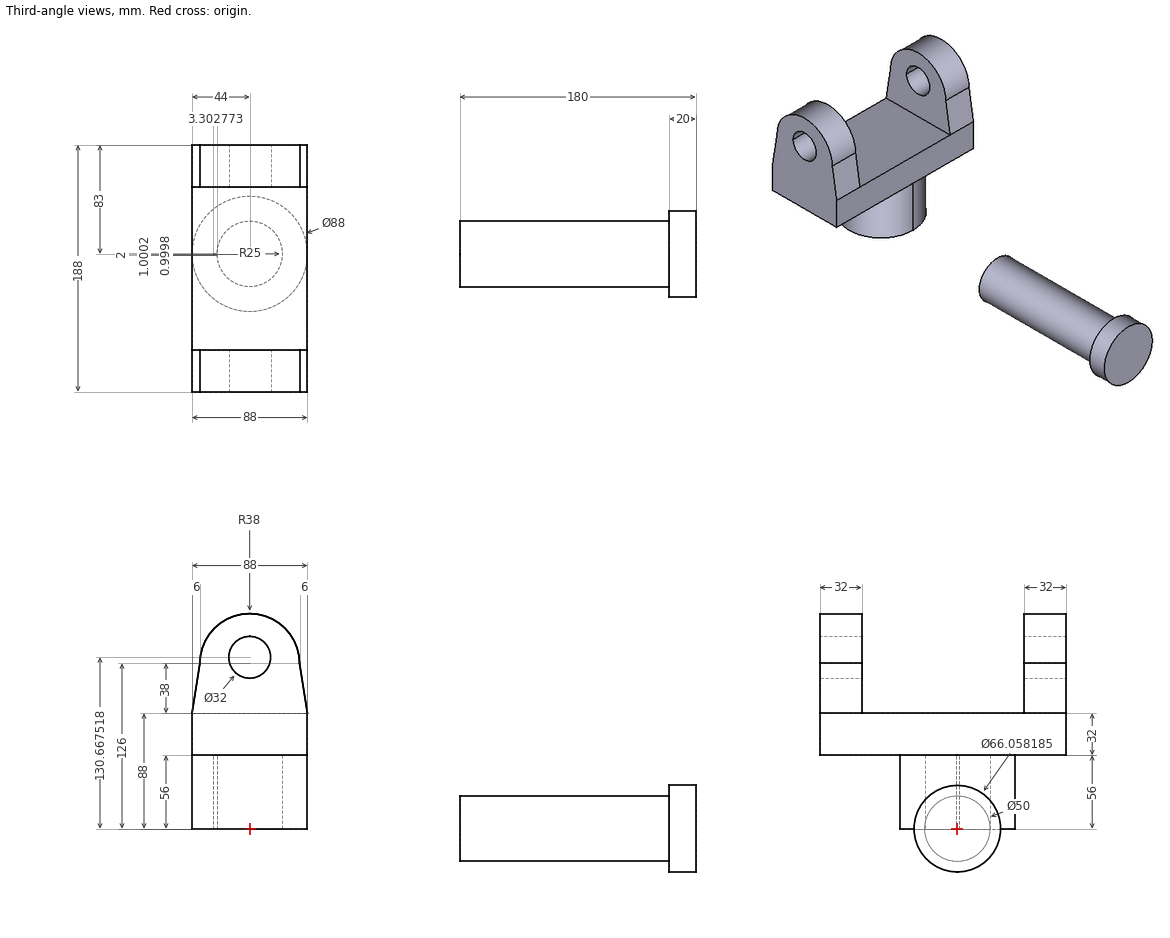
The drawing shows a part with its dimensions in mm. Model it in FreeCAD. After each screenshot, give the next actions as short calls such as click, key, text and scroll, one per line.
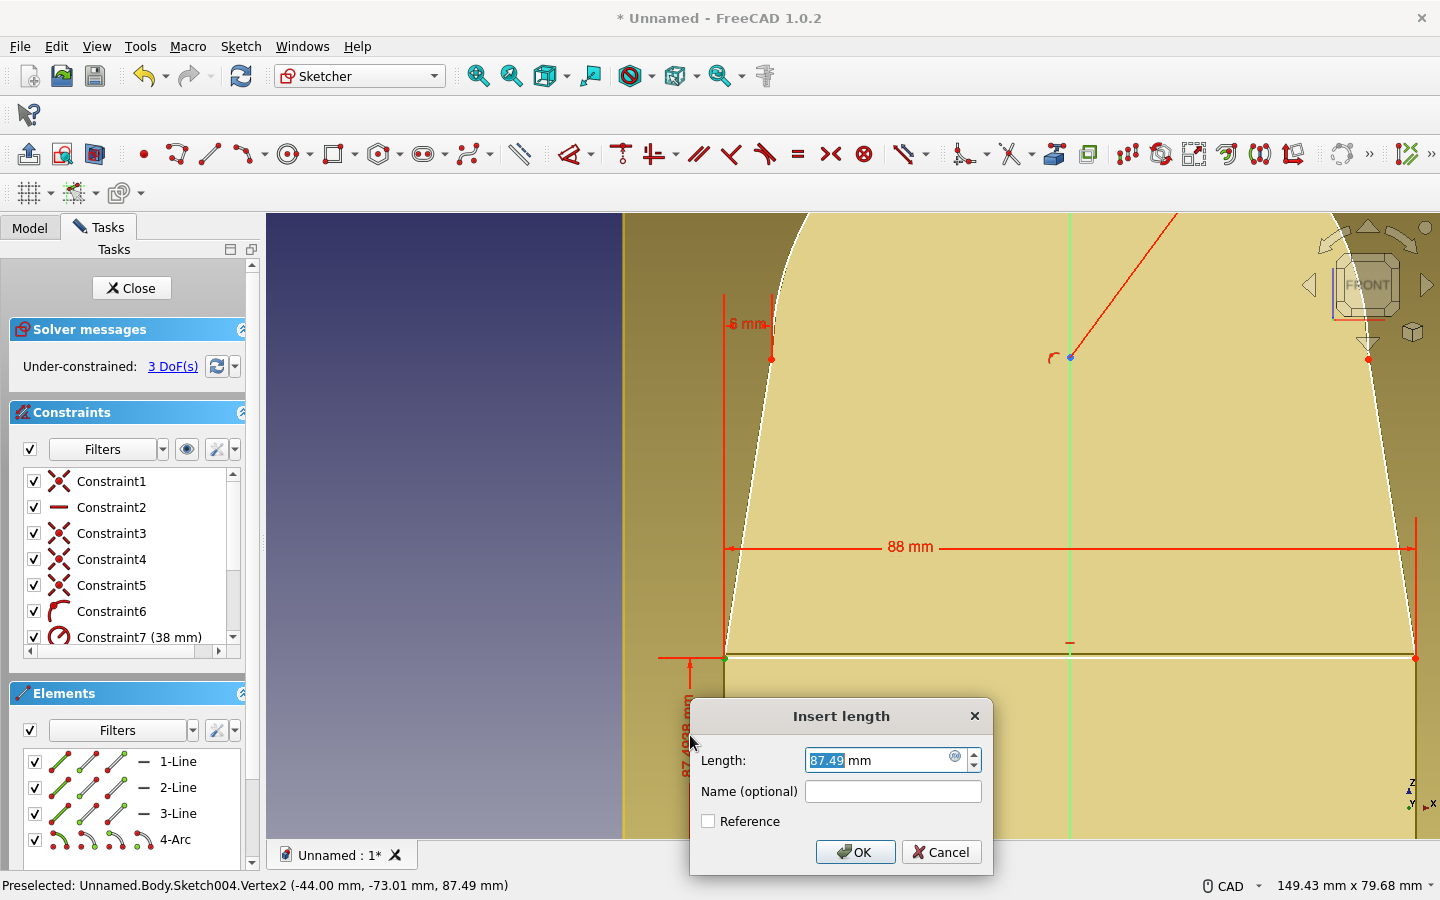
text(88)
key(Return)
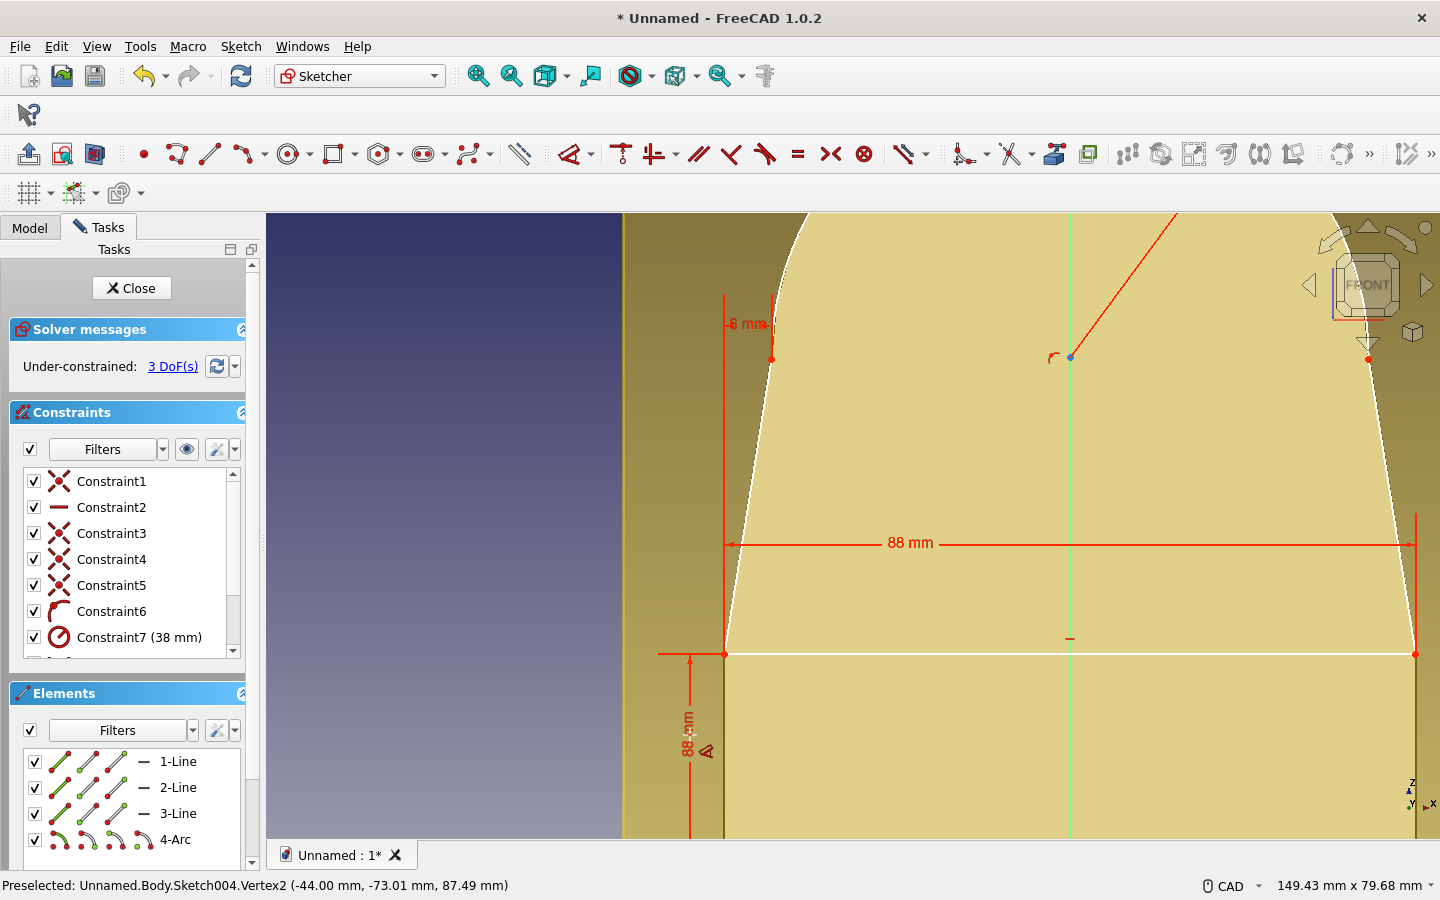
click(757, 448)
click(690, 507)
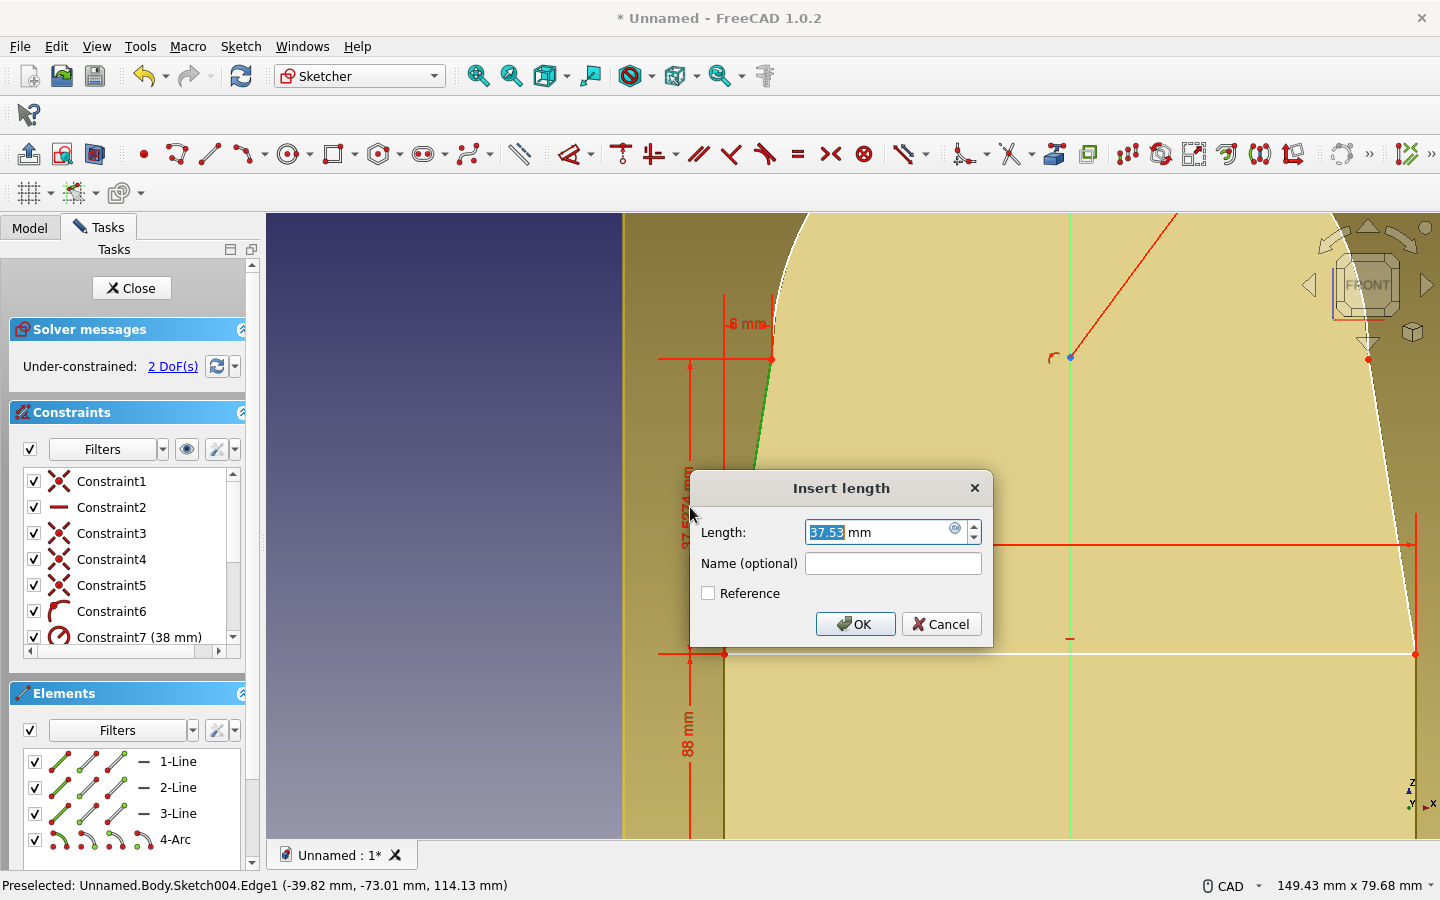
text(38)
key(Return)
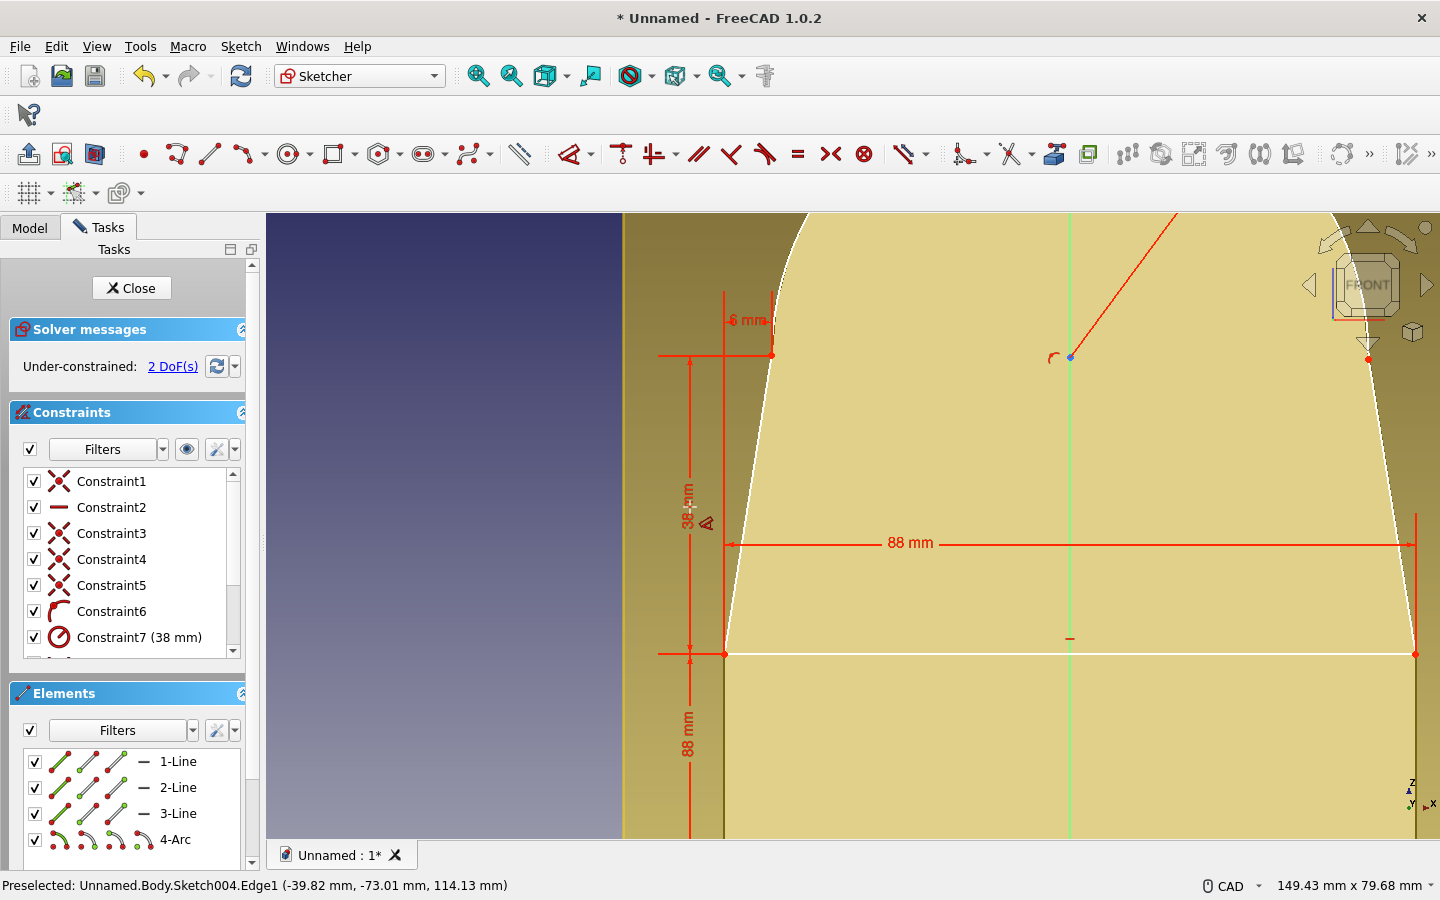
scroll(661, 450, down, 6)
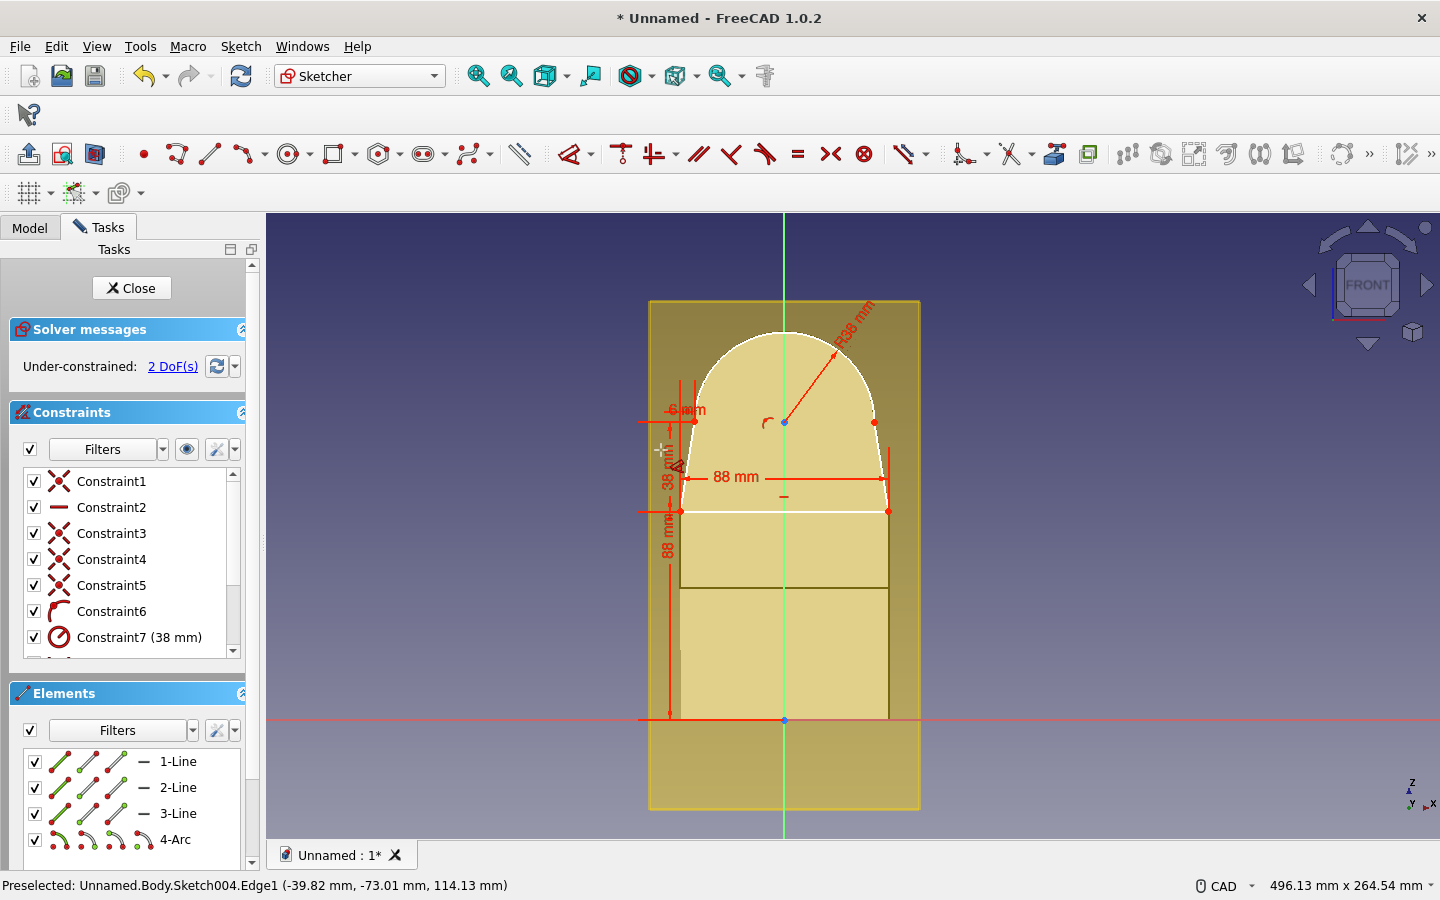
click(884, 485)
click(923, 467)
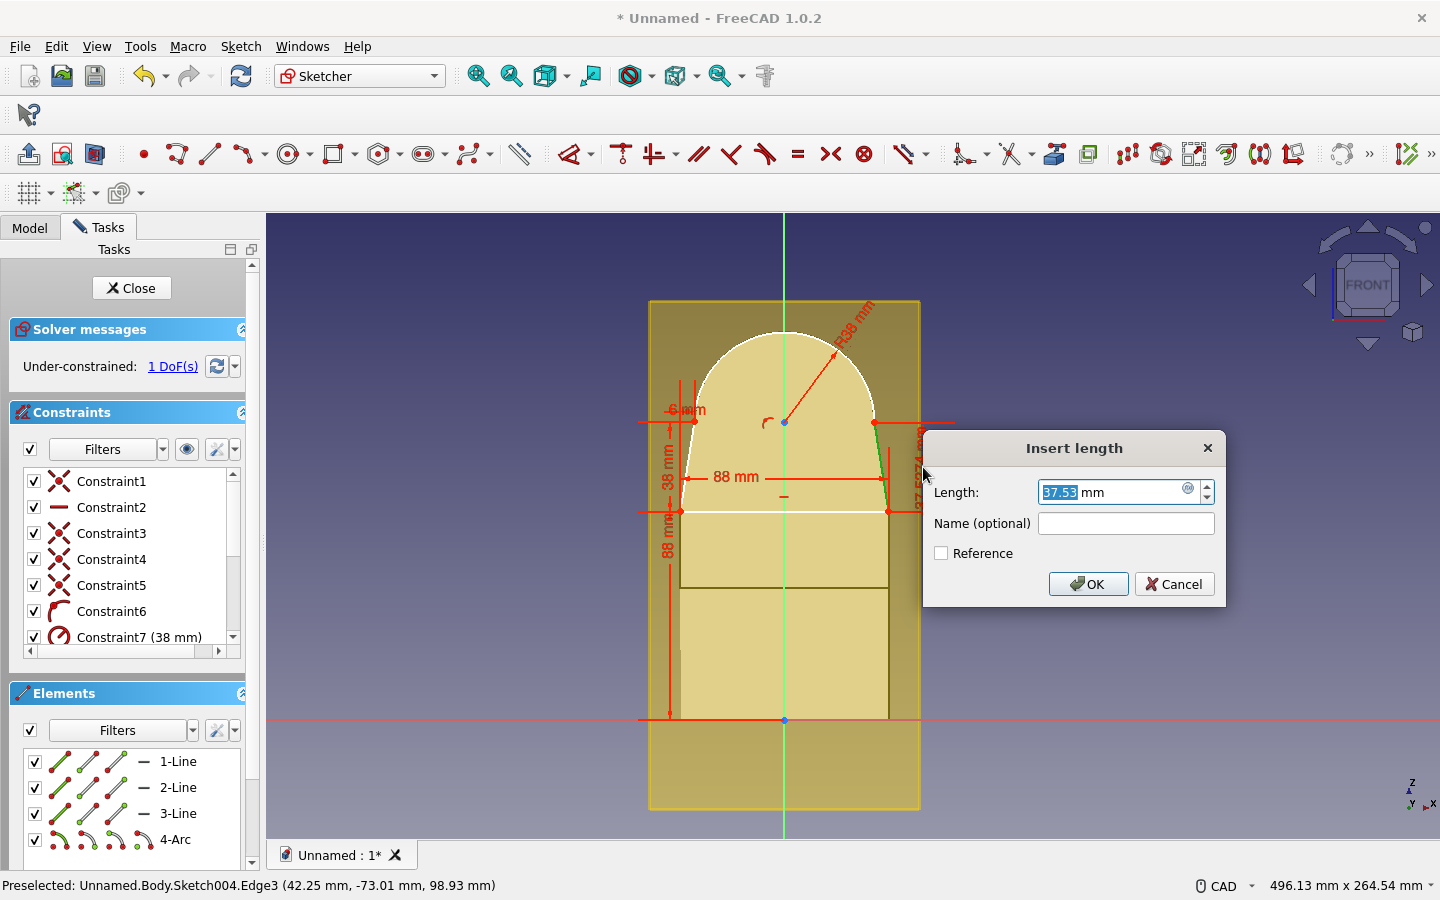
text(38)
key(Return)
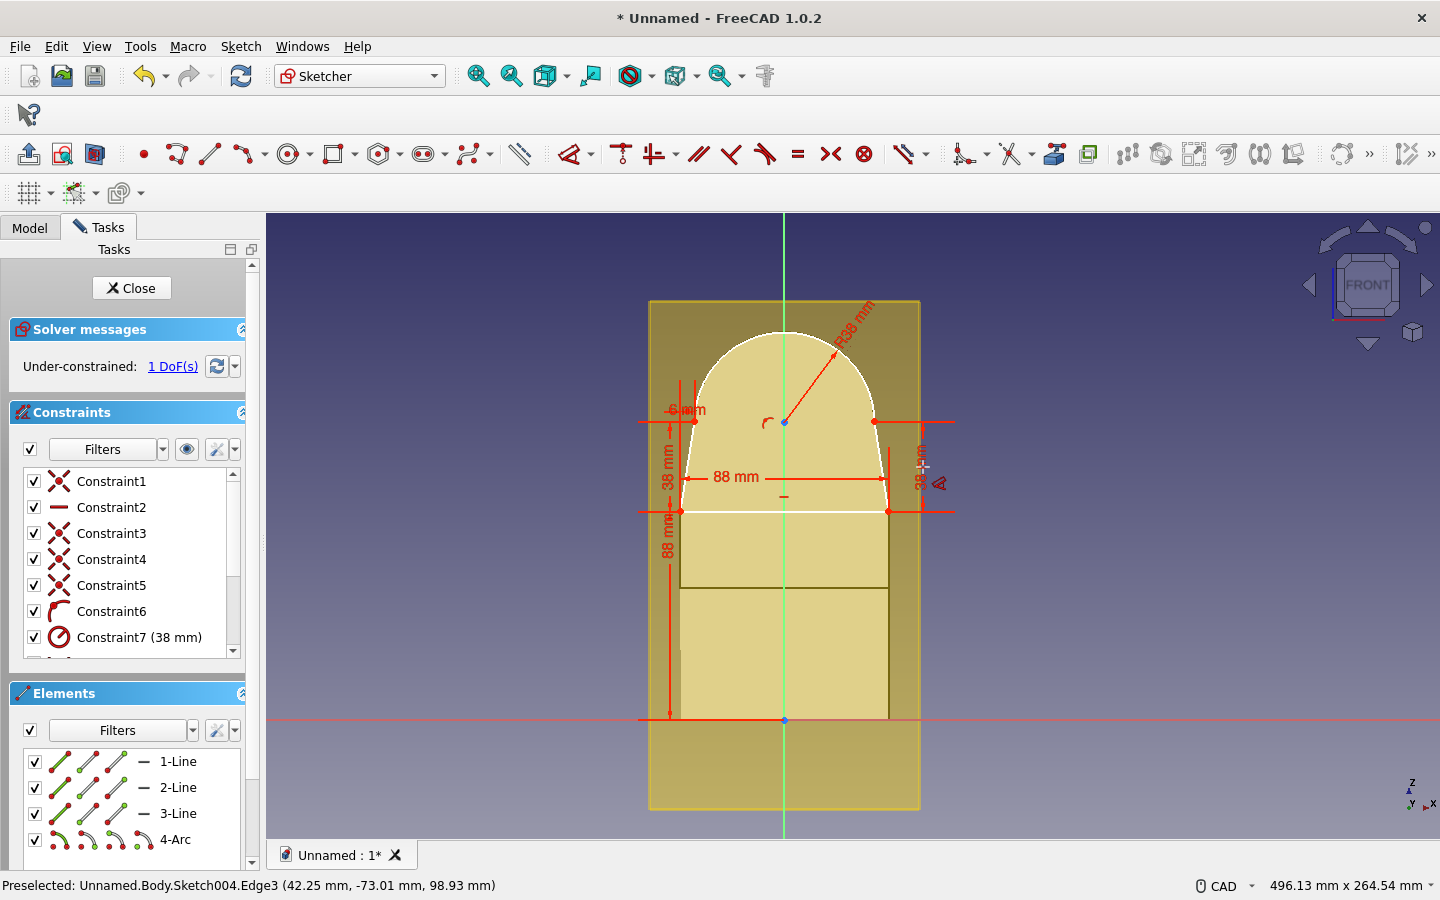
click(784, 423)
click(818, 571)